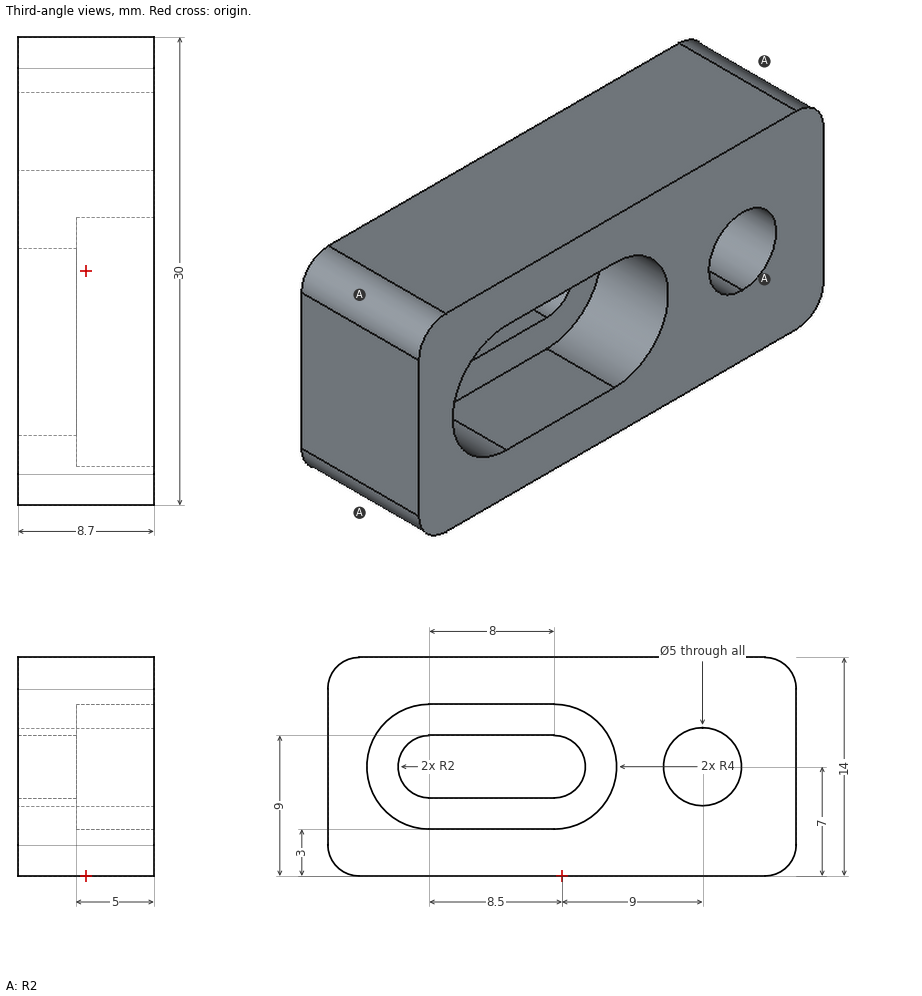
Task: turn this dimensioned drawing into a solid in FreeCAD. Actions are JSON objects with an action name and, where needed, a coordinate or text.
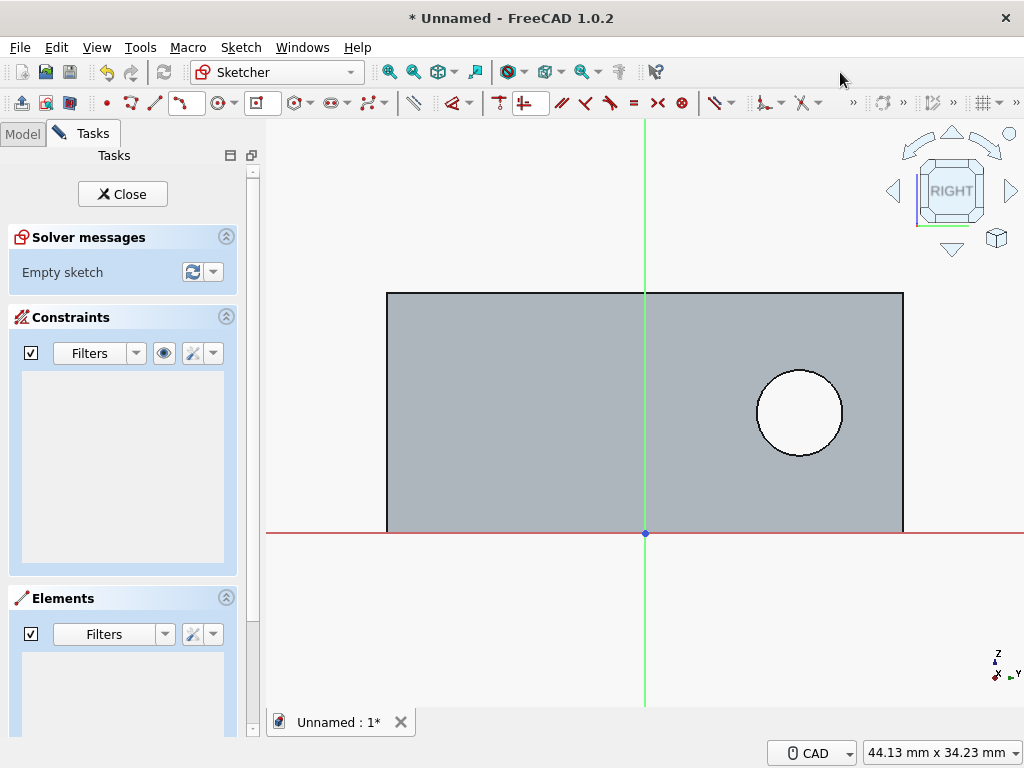
{"action": "scroll", "coordinate": [557, 508], "scroll_direction": "up", "scroll_amount": 3}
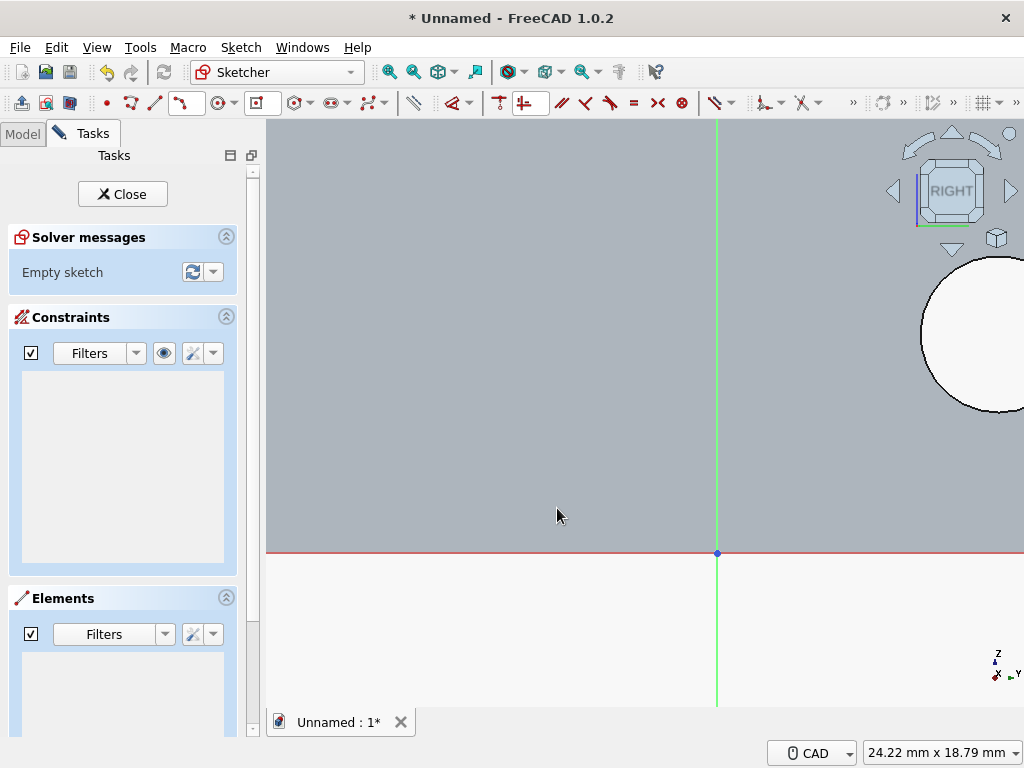
{"action": "left_click", "coordinate": [332, 104]}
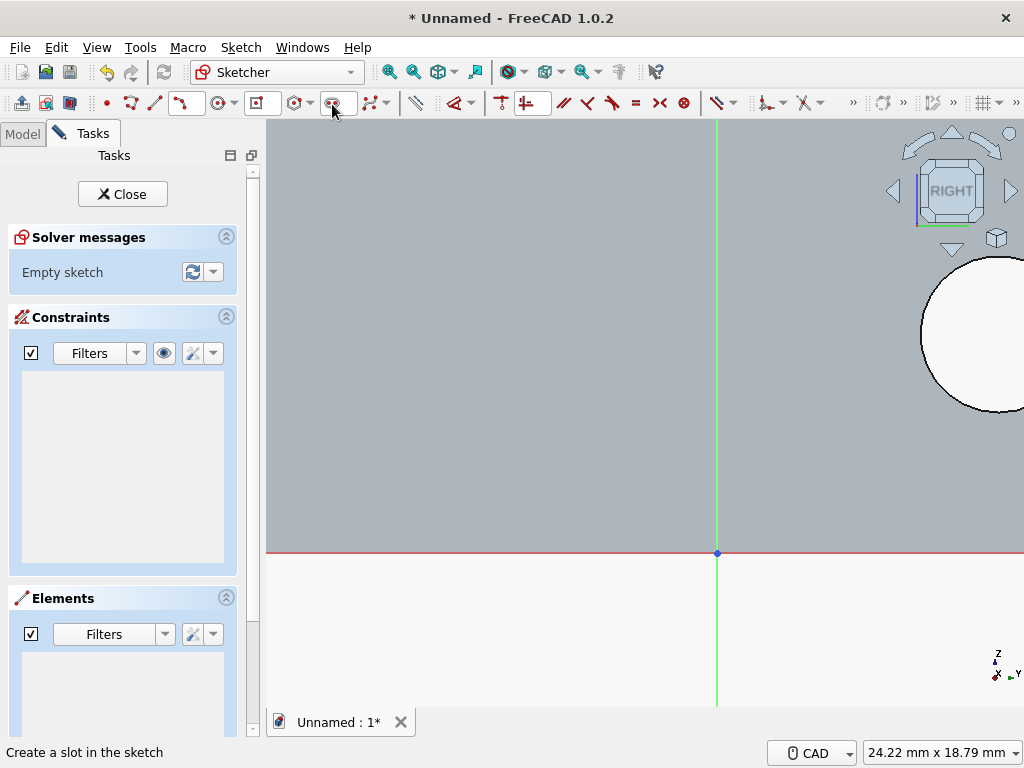
{"action": "left_click", "coordinate": [451, 334]}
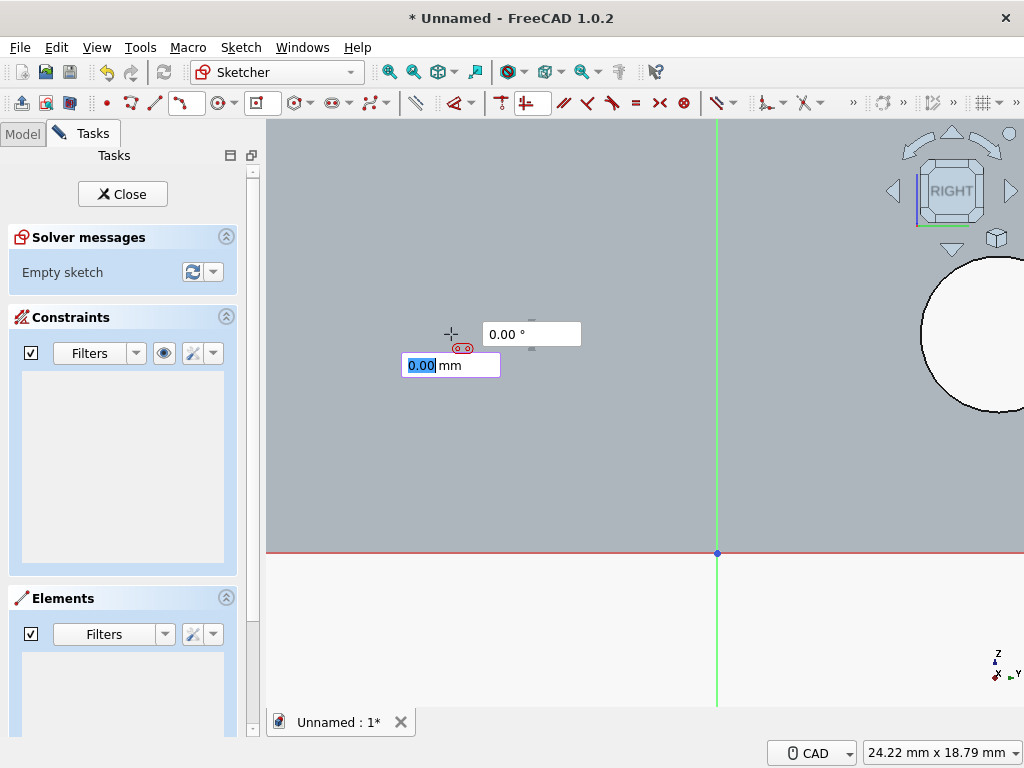
{"action": "left_click", "coordinate": [701, 334]}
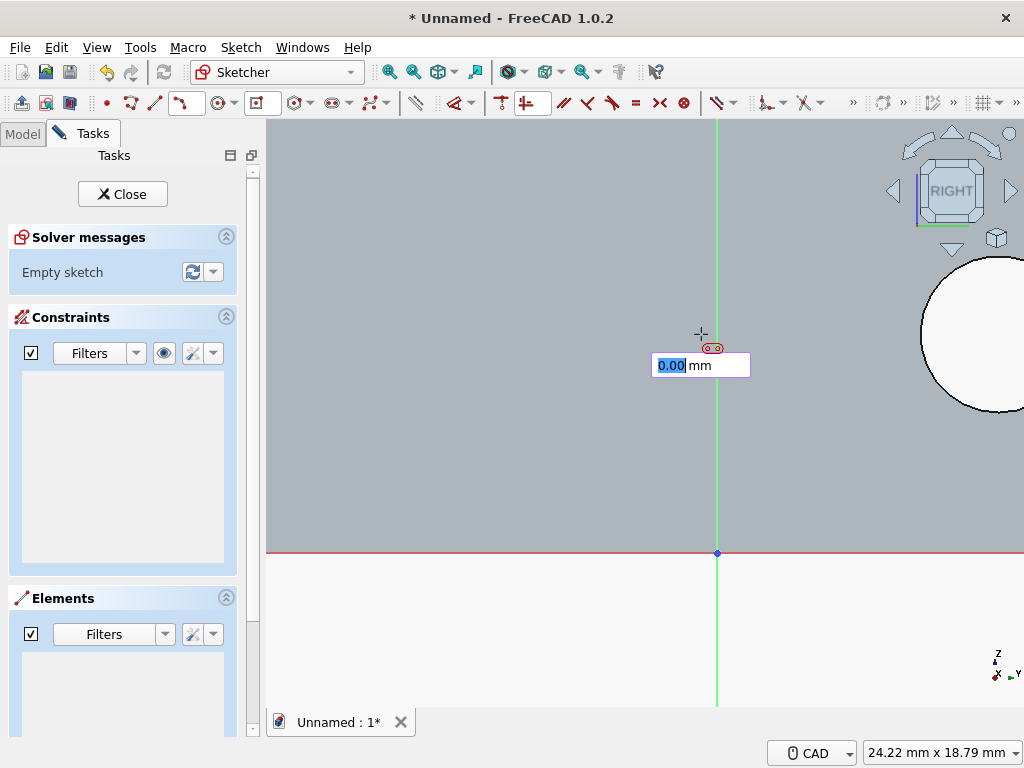
{"action": "left_click", "coordinate": [576, 272]}
{"action": "key", "text": "Escape"}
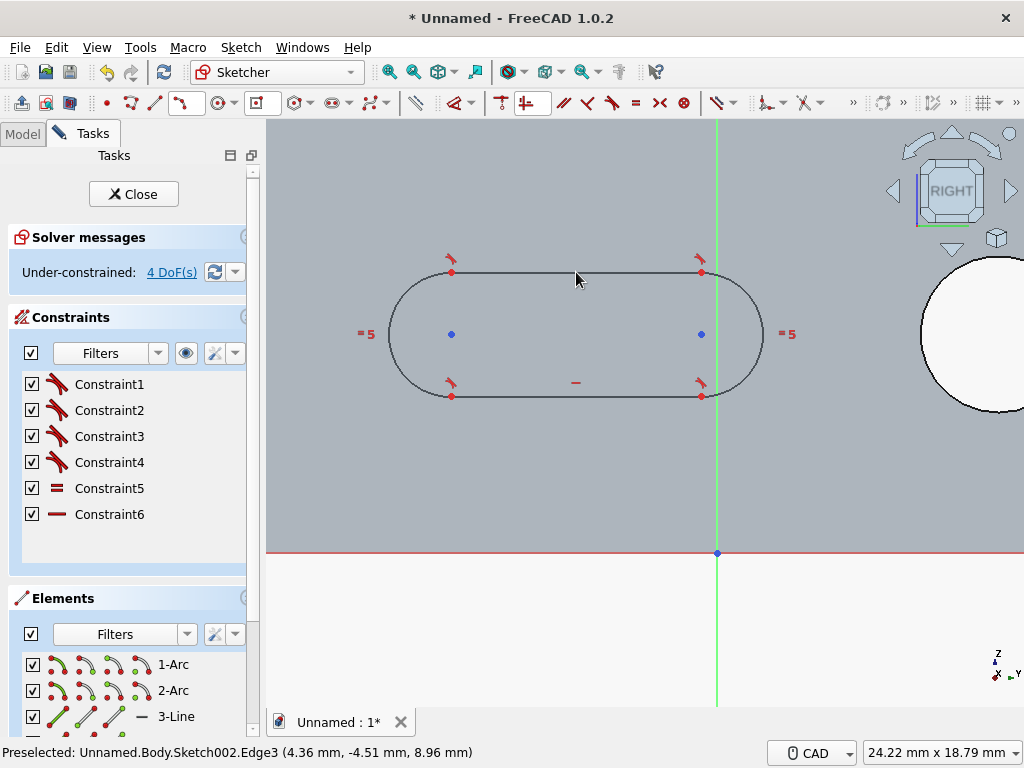
{"action": "left_click", "coordinate": [454, 104]}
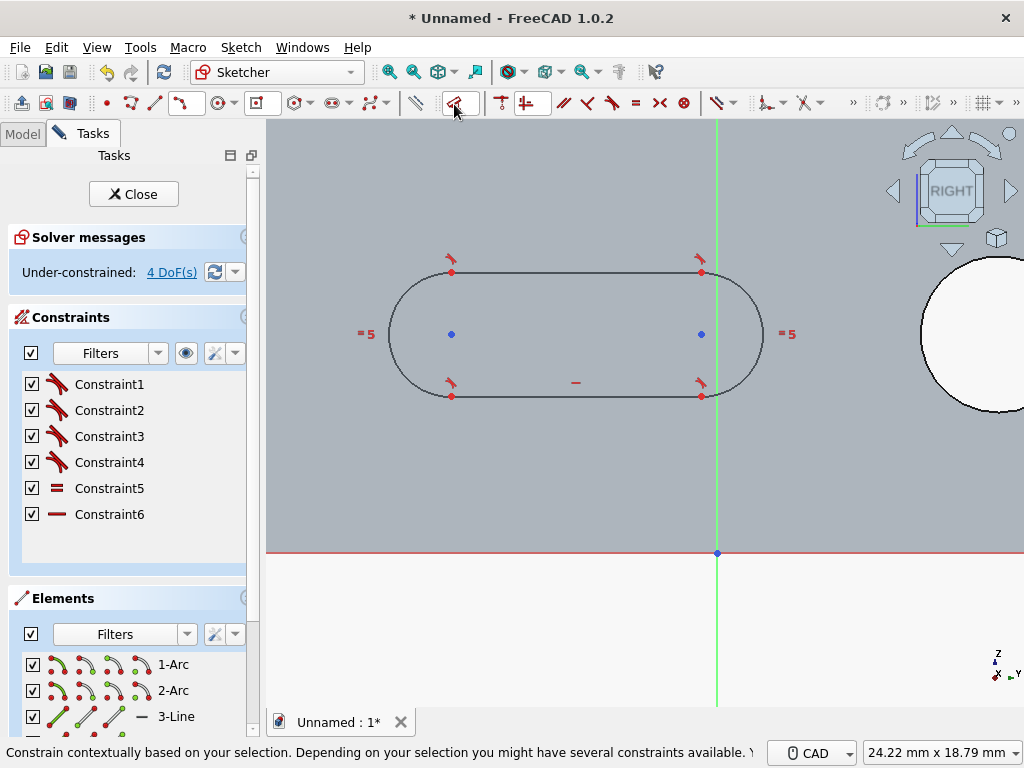
{"action": "left_click", "coordinate": [401, 299]}
{"action": "left_click", "coordinate": [375, 280]}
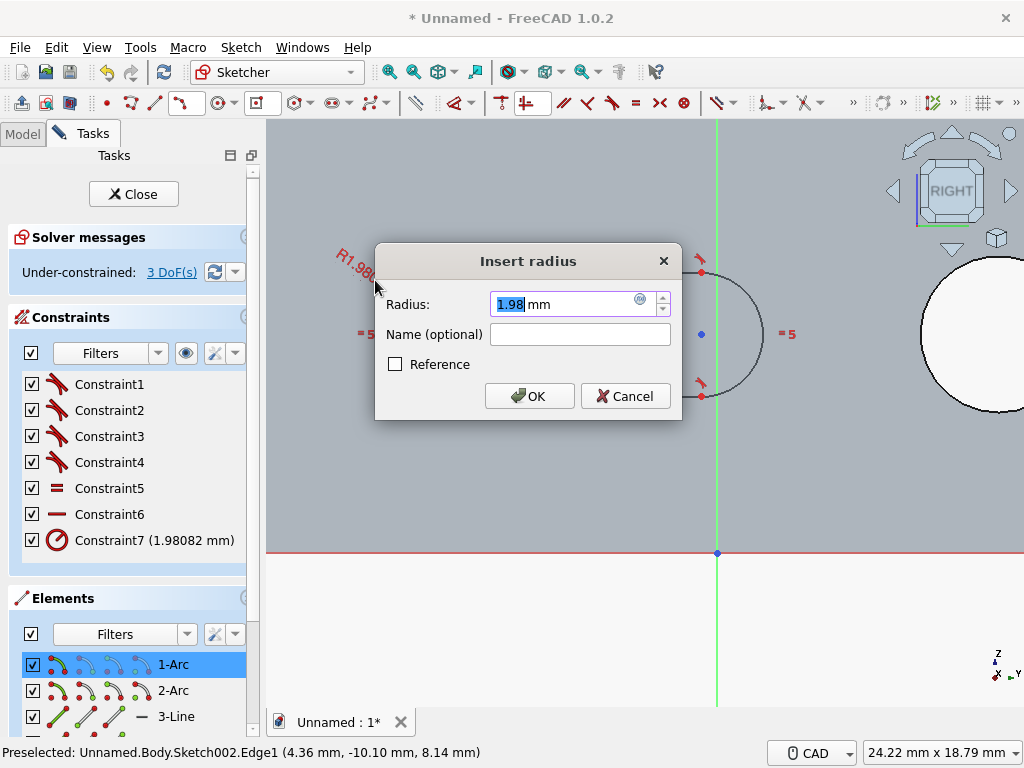
{"action": "type", "text": "2"}
{"action": "key", "text": "Return"}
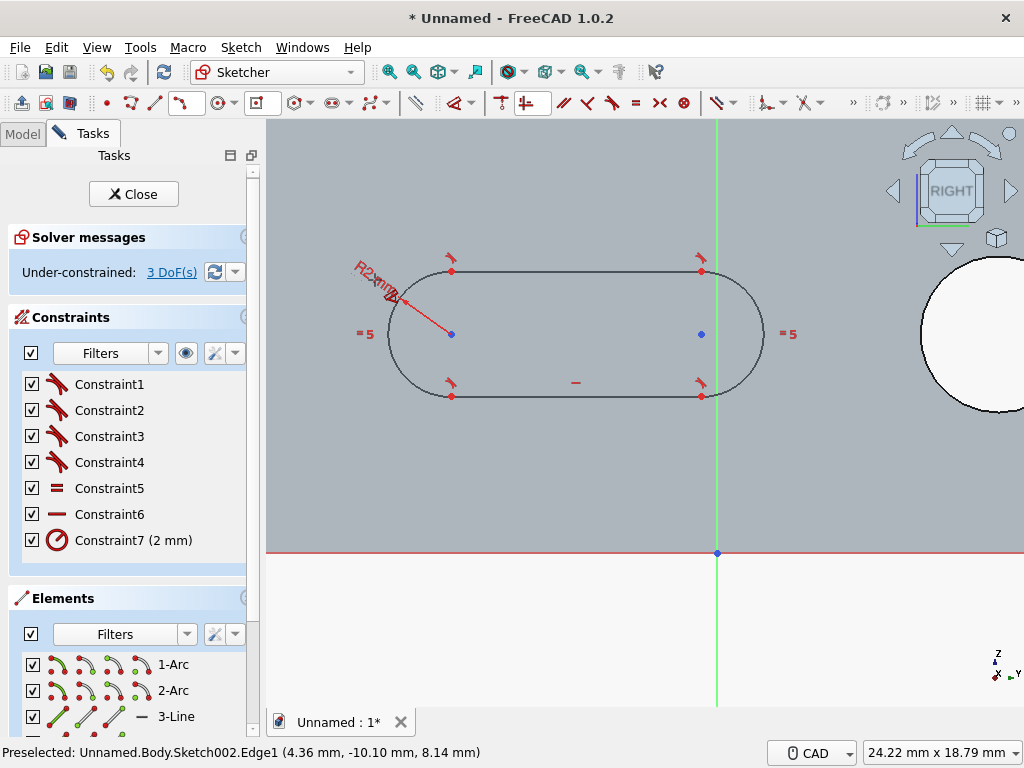
{"action": "left_click", "coordinate": [526, 272]}
{"action": "left_click", "coordinate": [576, 238]}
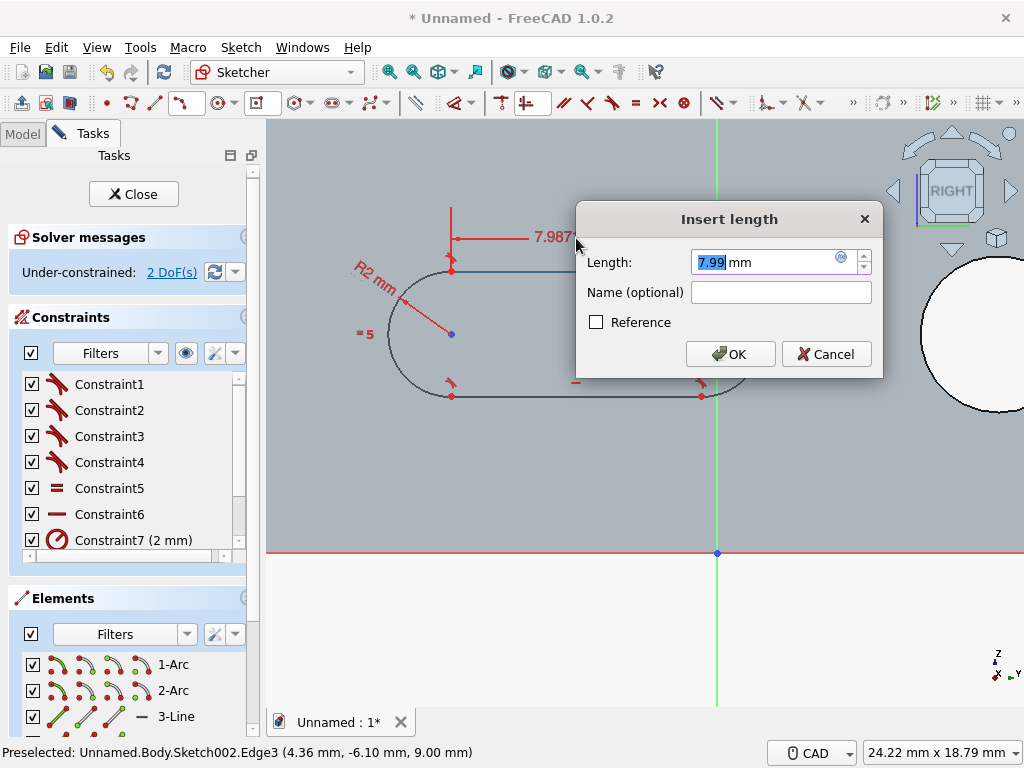
{"action": "type", "text": "8"}
{"action": "key", "text": "Return"}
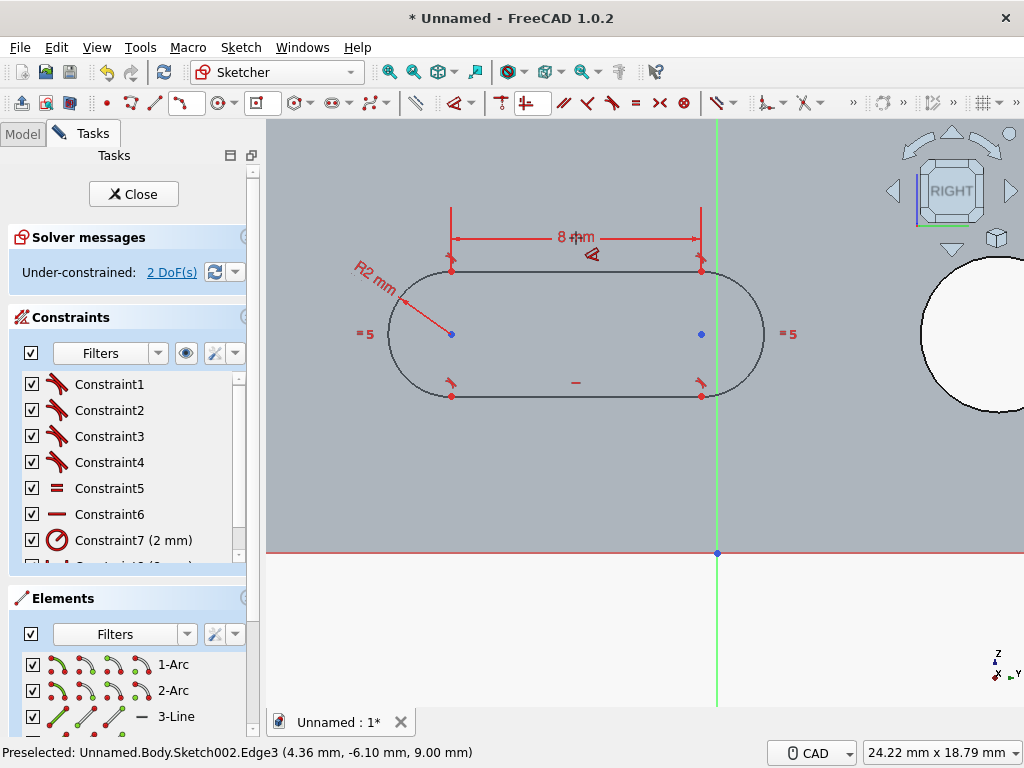
{"action": "left_click", "coordinate": [451, 272]}
{"action": "left_click", "coordinate": [751, 413]}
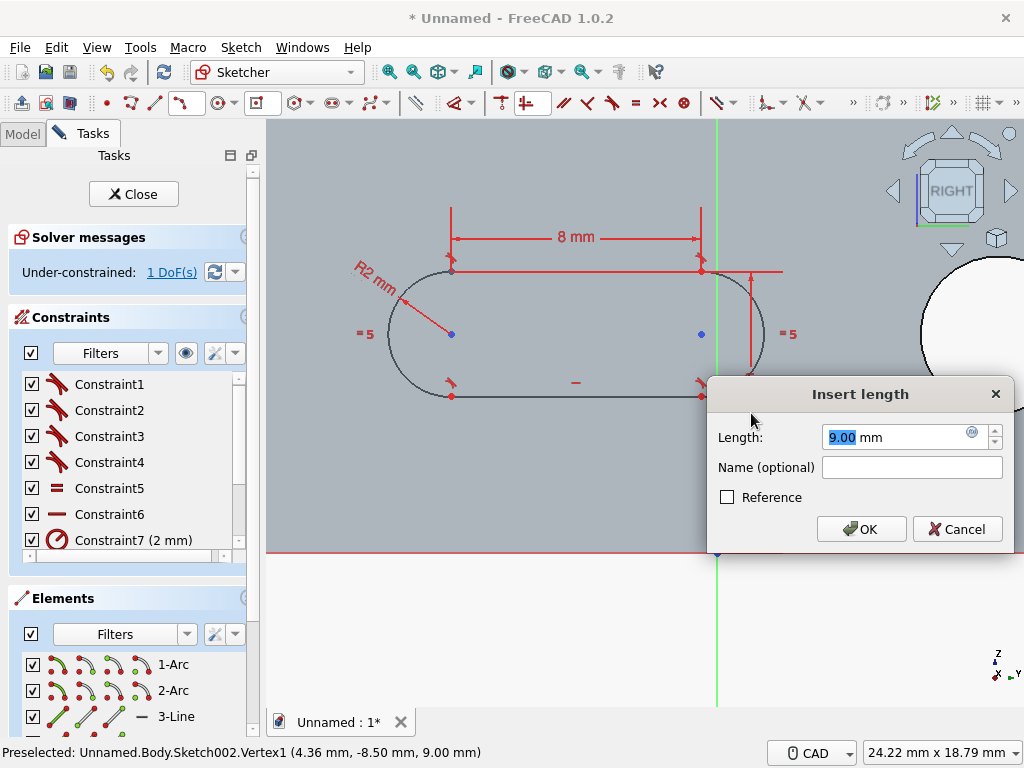
{"action": "type", "text": "9"}
{"action": "key", "text": "Return"}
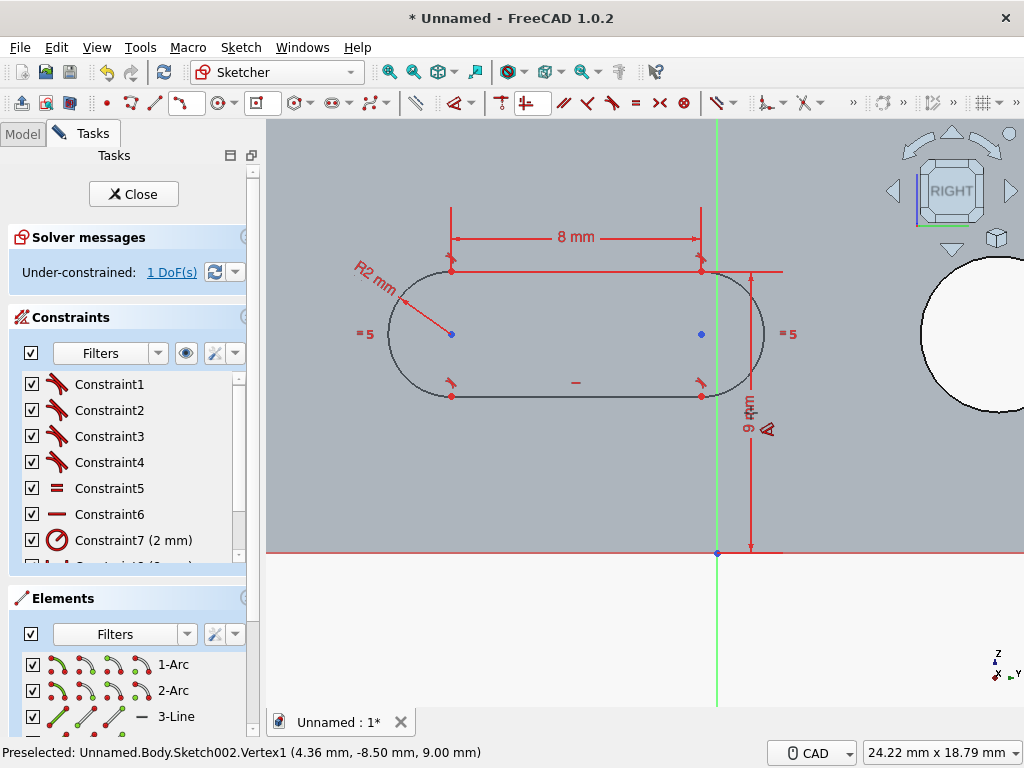
{"action": "left_click", "coordinate": [451, 272]}
{"action": "left_click", "coordinate": [584, 587]}